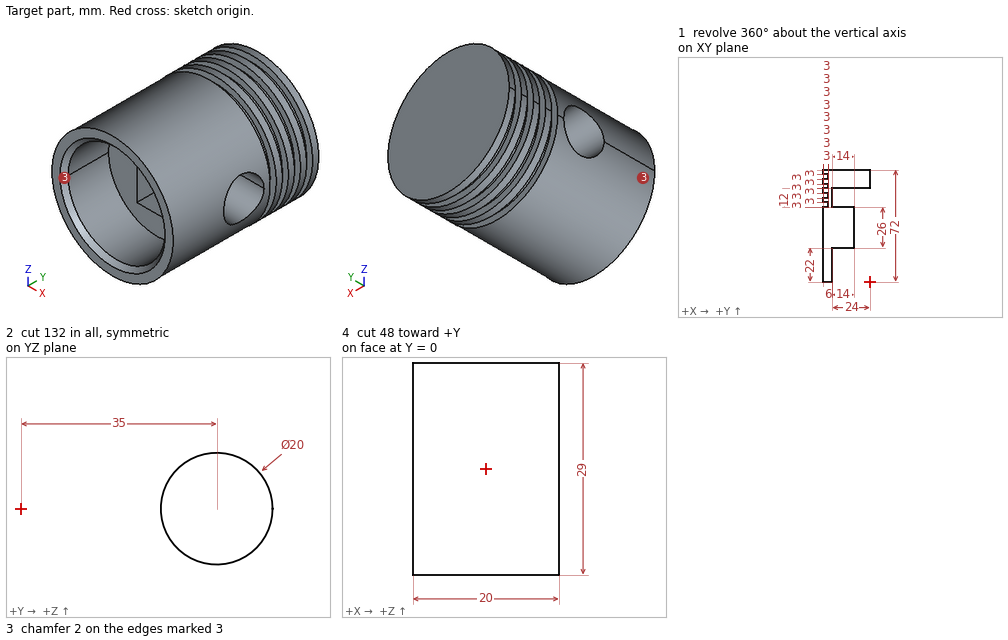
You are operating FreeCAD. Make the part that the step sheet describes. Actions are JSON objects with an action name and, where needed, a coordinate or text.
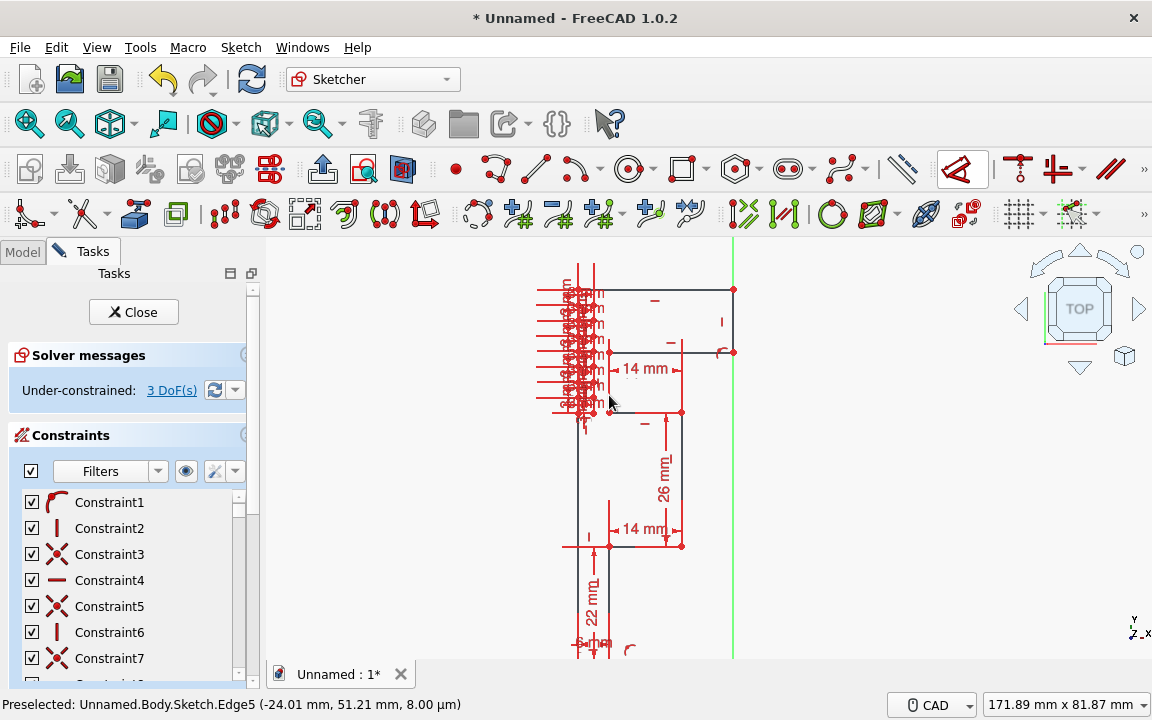
{"action": "key", "text": "i"}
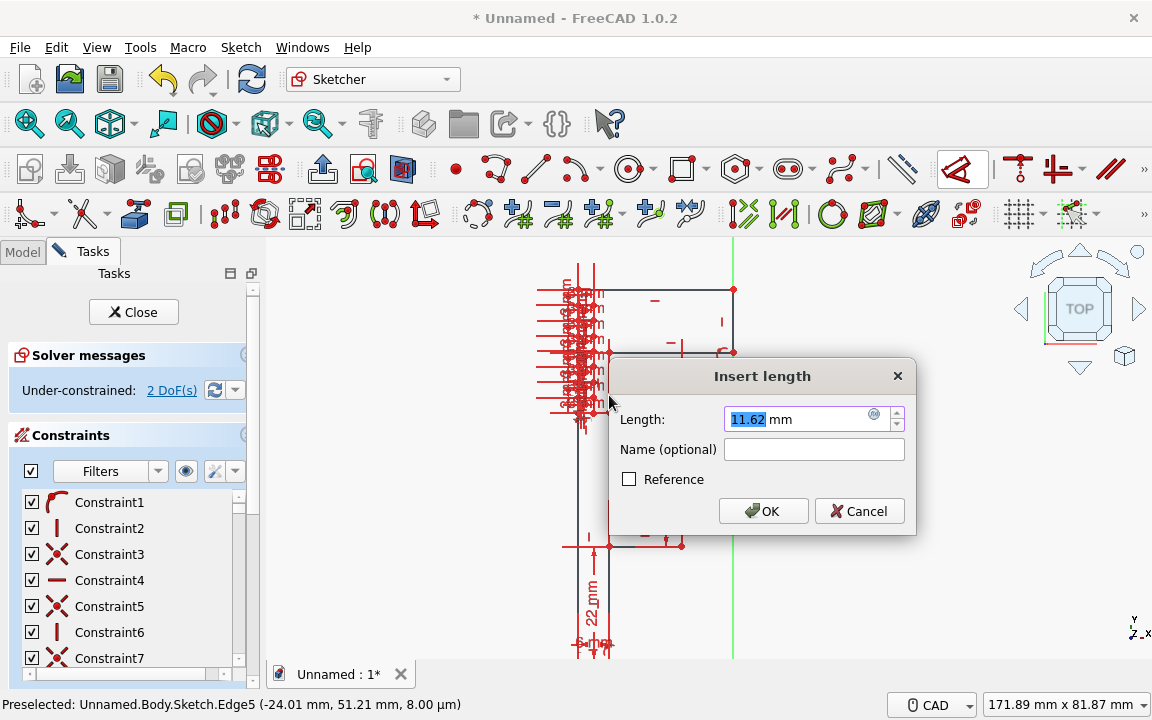
{"action": "type", "text": "12"}
{"action": "key", "text": "Return"}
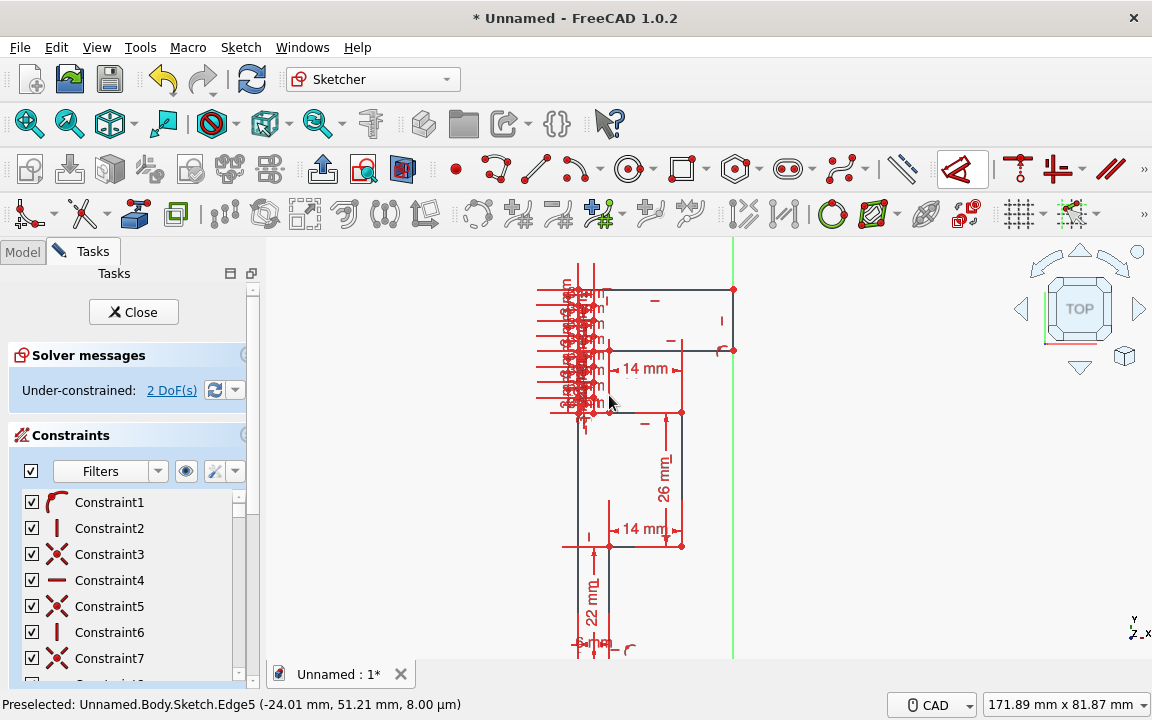
{"action": "scroll", "coordinate": [609, 394], "scroll_direction": "down", "scroll_amount": 2}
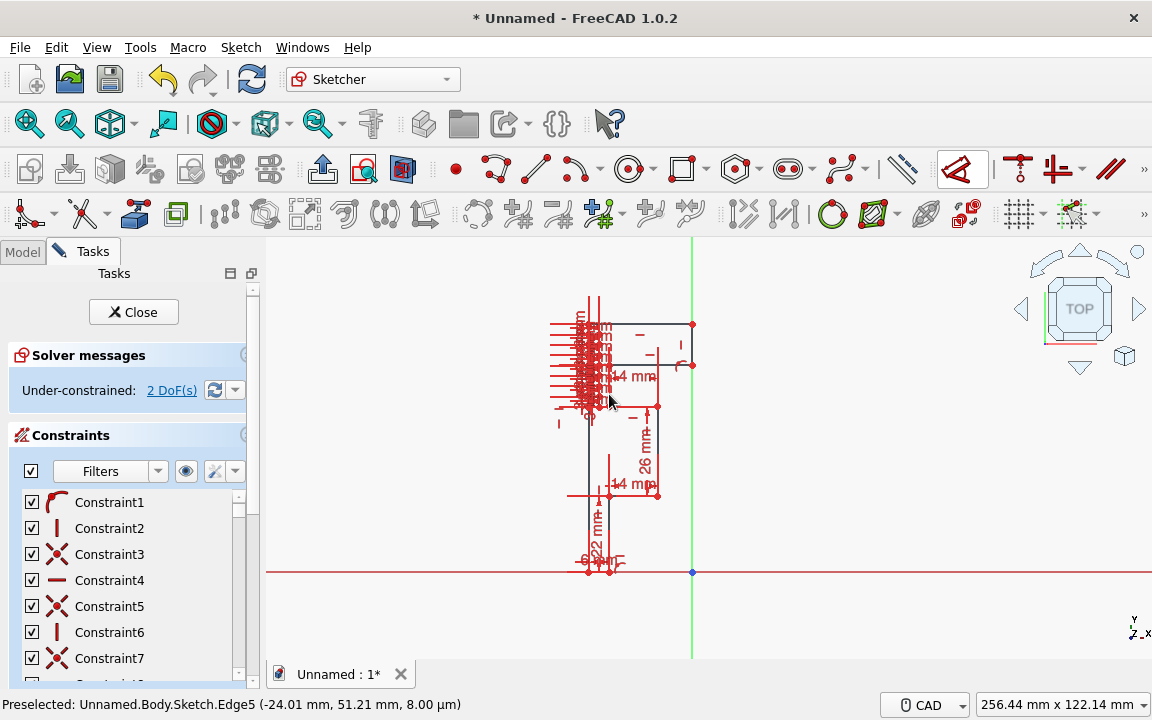
{"action": "left_click", "coordinate": [609, 572]}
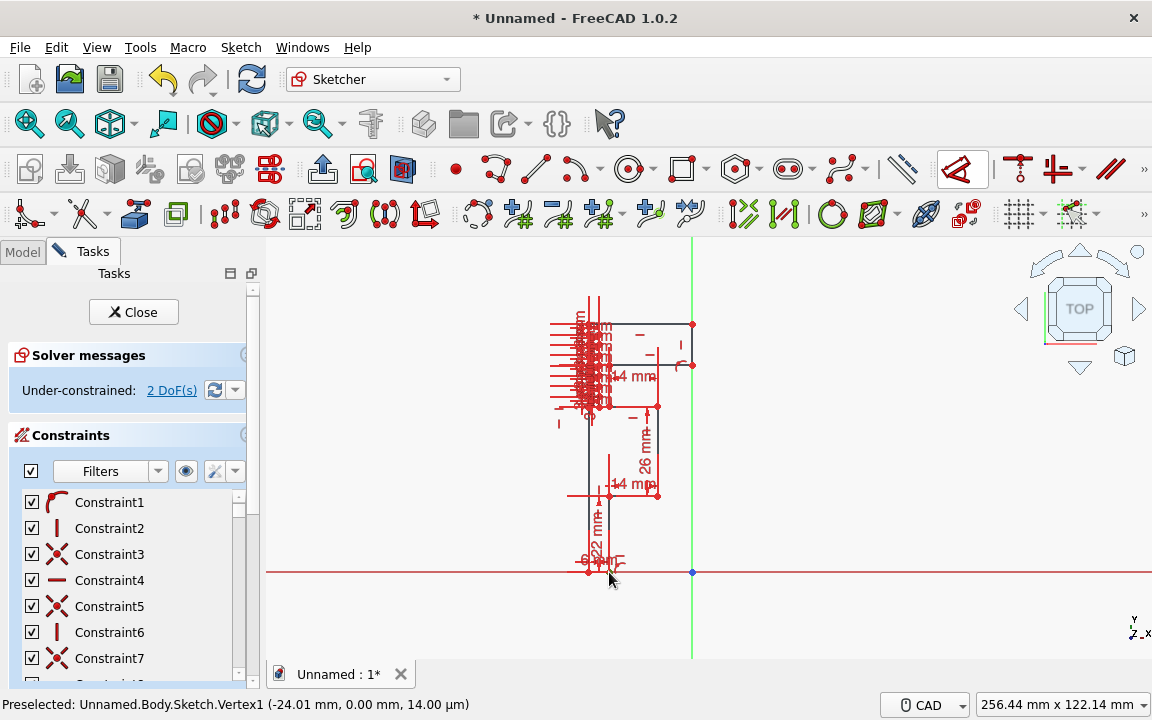
{"action": "key", "text": "l"}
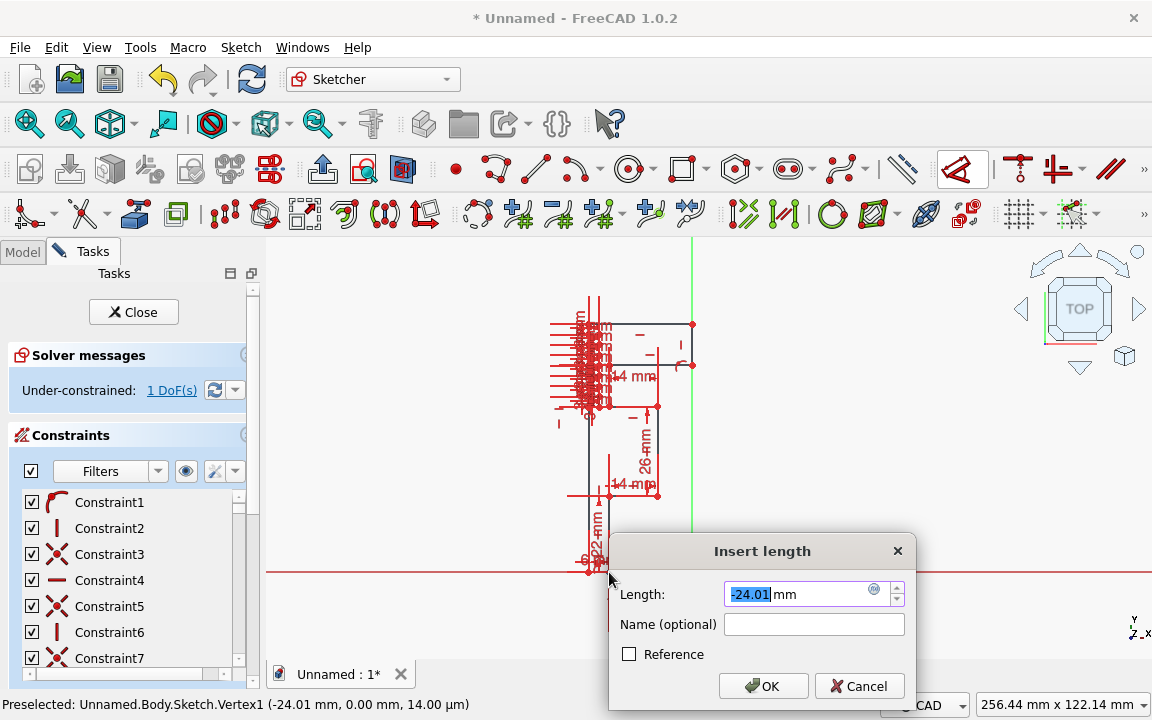
{"action": "type", "text": "-24"}
{"action": "key", "text": "Return"}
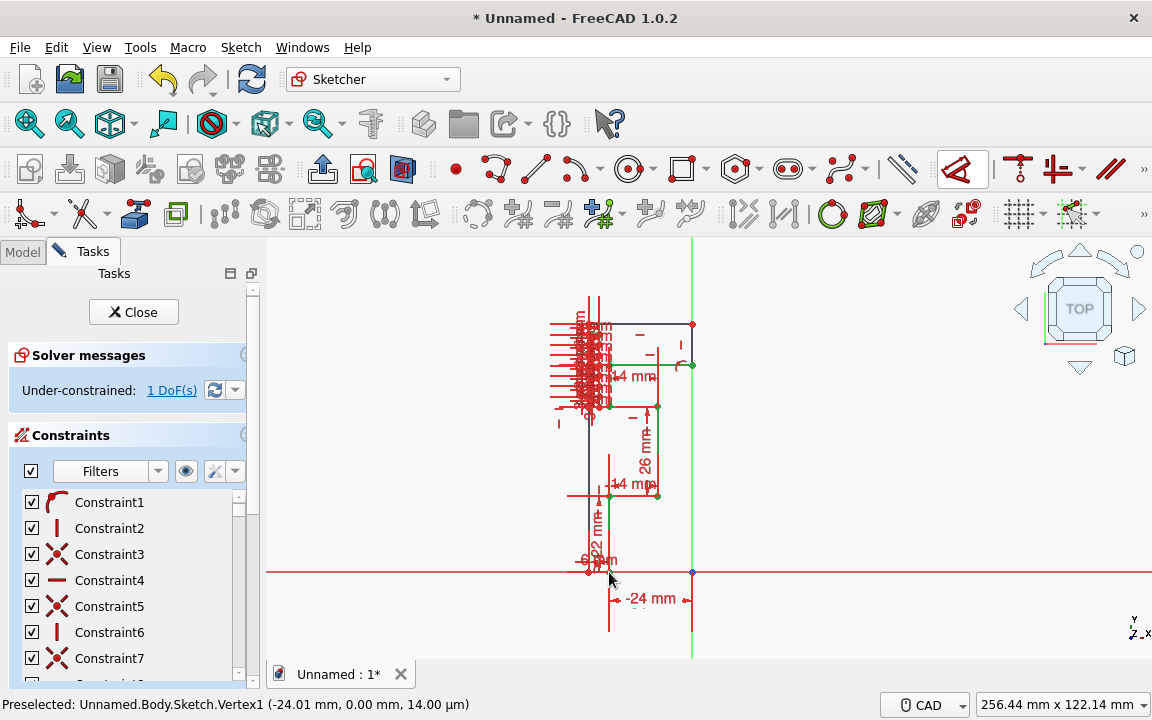
{"action": "left_click", "coordinate": [692, 324]}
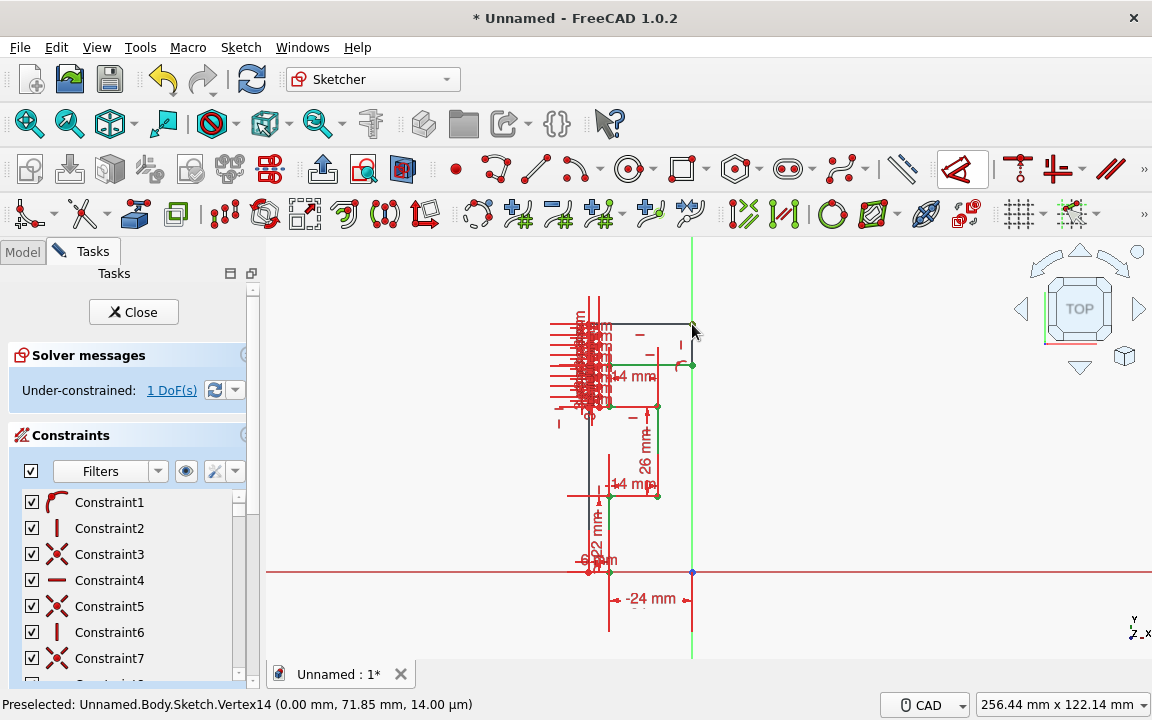
{"action": "left_click", "coordinate": [982, 170]}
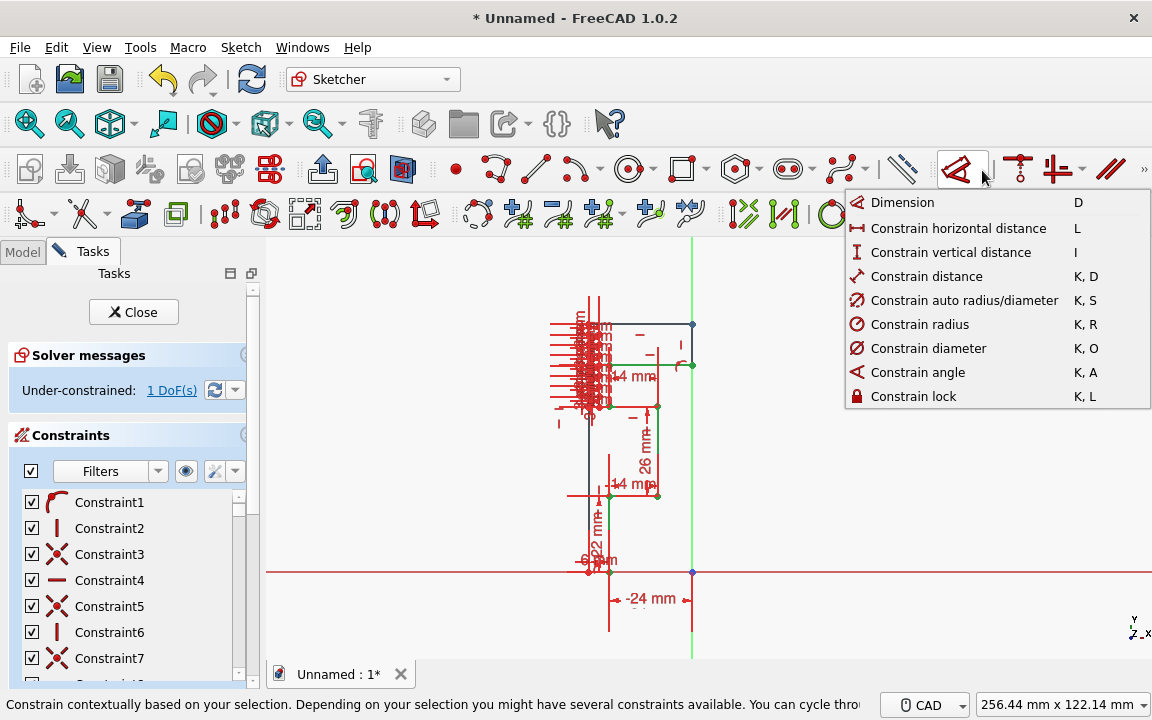
{"action": "left_click", "coordinate": [998, 252]}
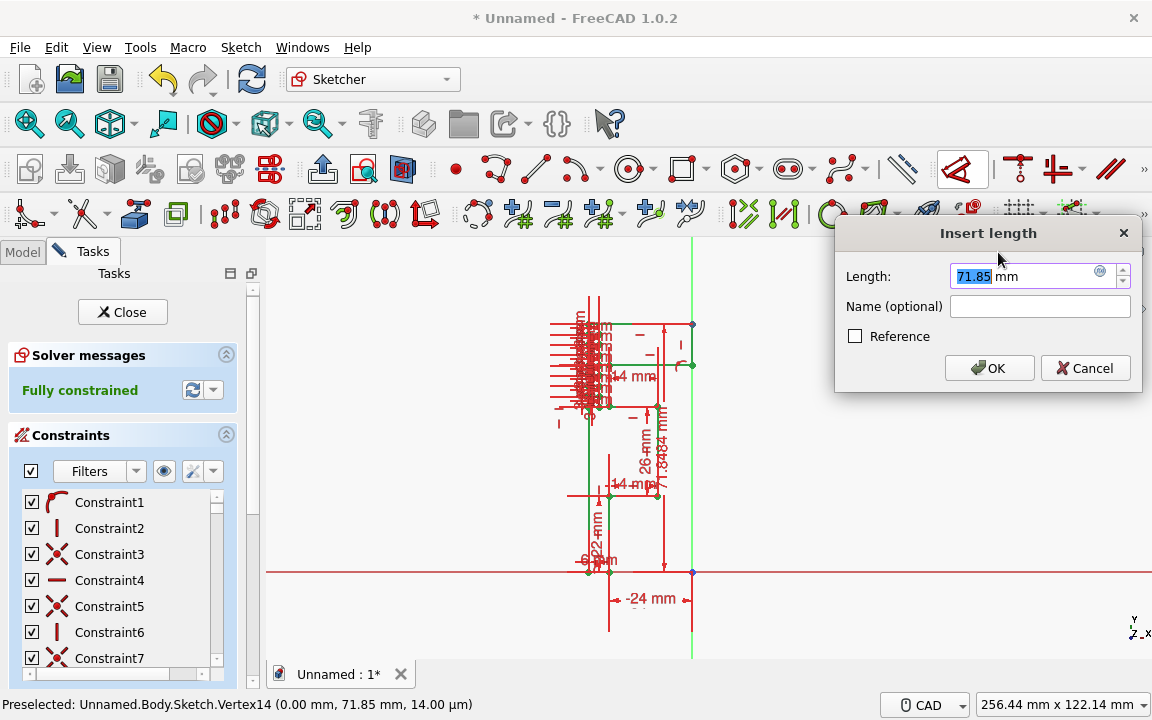
{"action": "type", "text": "72"}
{"action": "key", "text": "Return"}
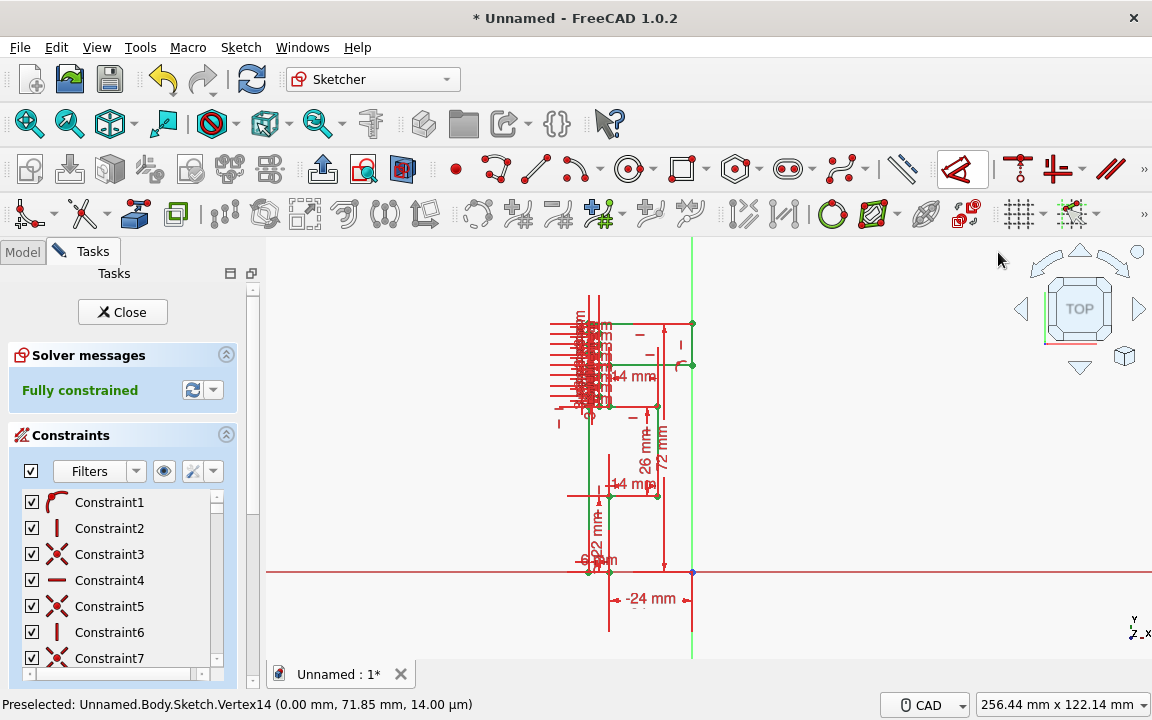
{"action": "left_click", "coordinate": [123, 312]}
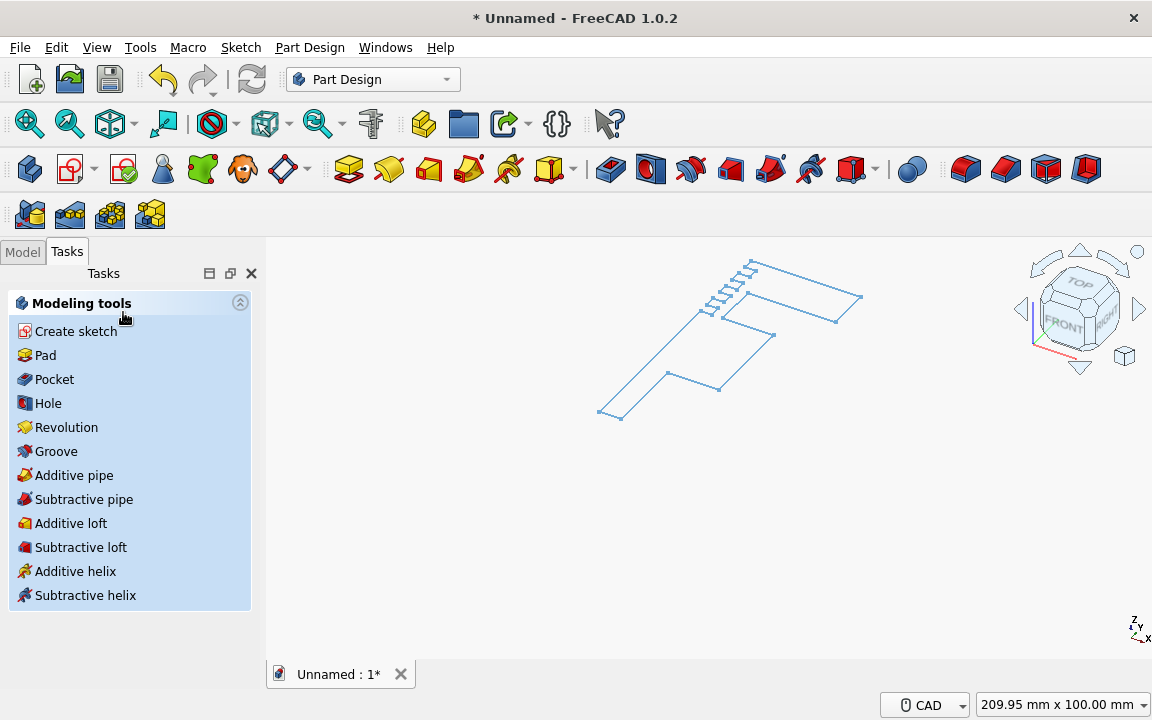
{"action": "left_click", "coordinate": [390, 170]}